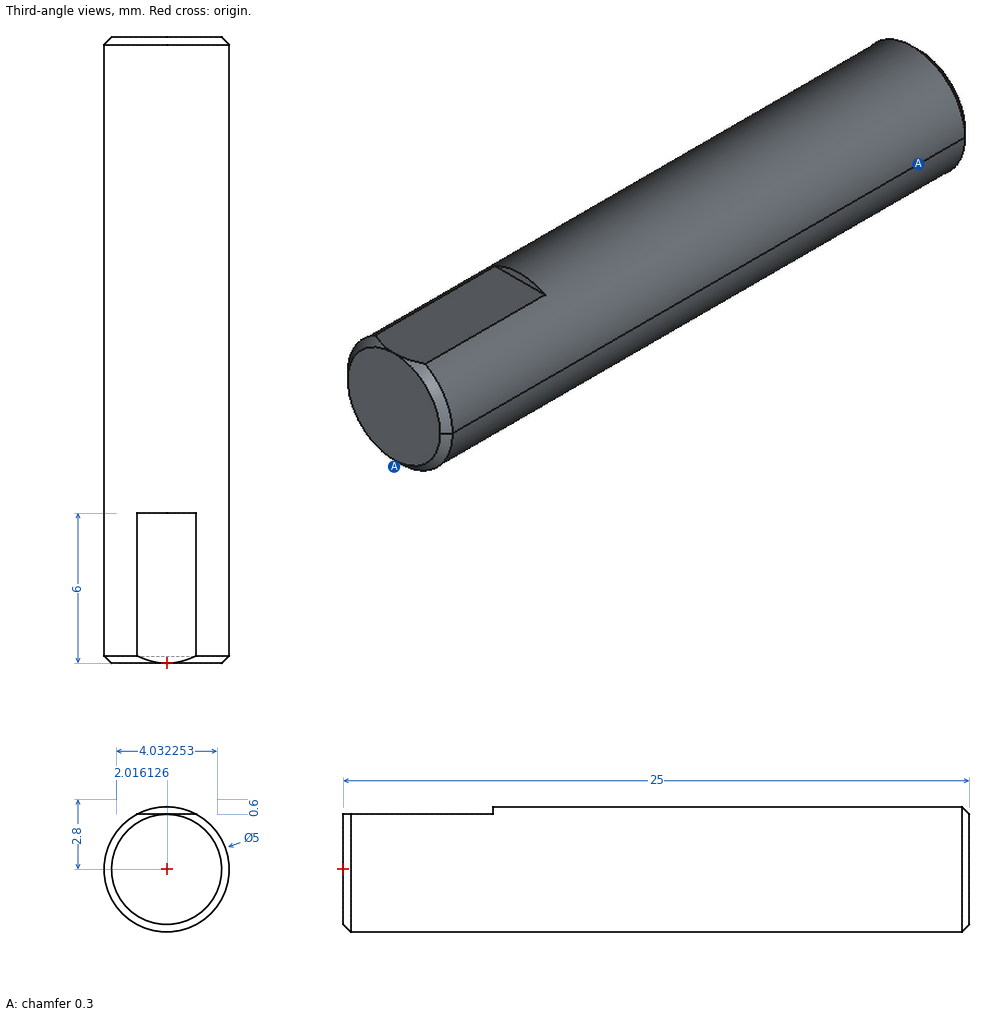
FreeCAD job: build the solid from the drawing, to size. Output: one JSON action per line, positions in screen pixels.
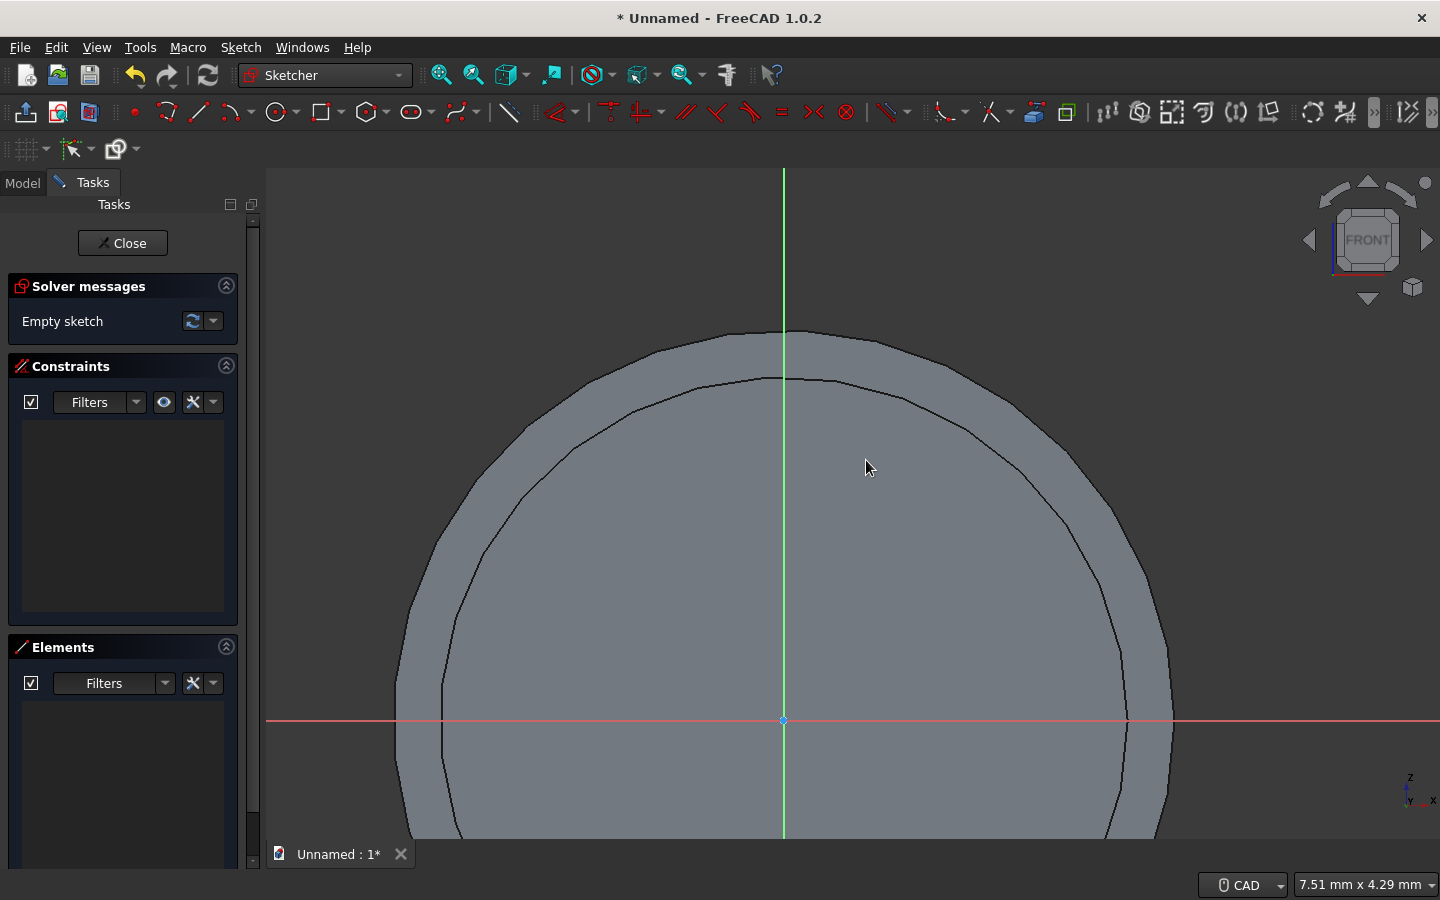
{"action": "left_click", "coordinate": [322, 112]}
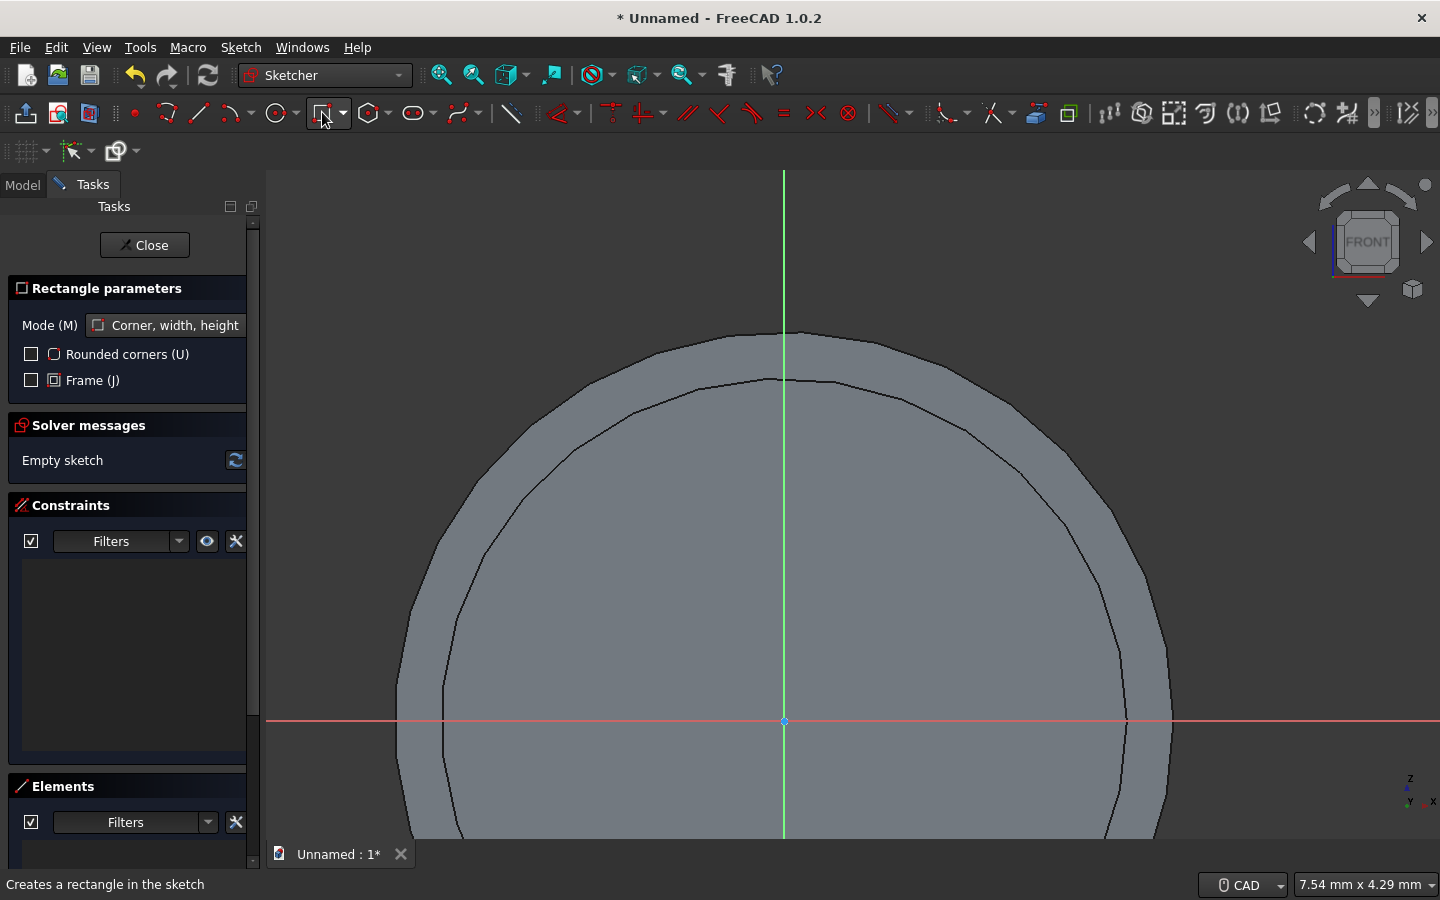
{"action": "left_click", "coordinate": [470, 285]}
{"action": "mouse_move", "coordinate": [1098, 379]}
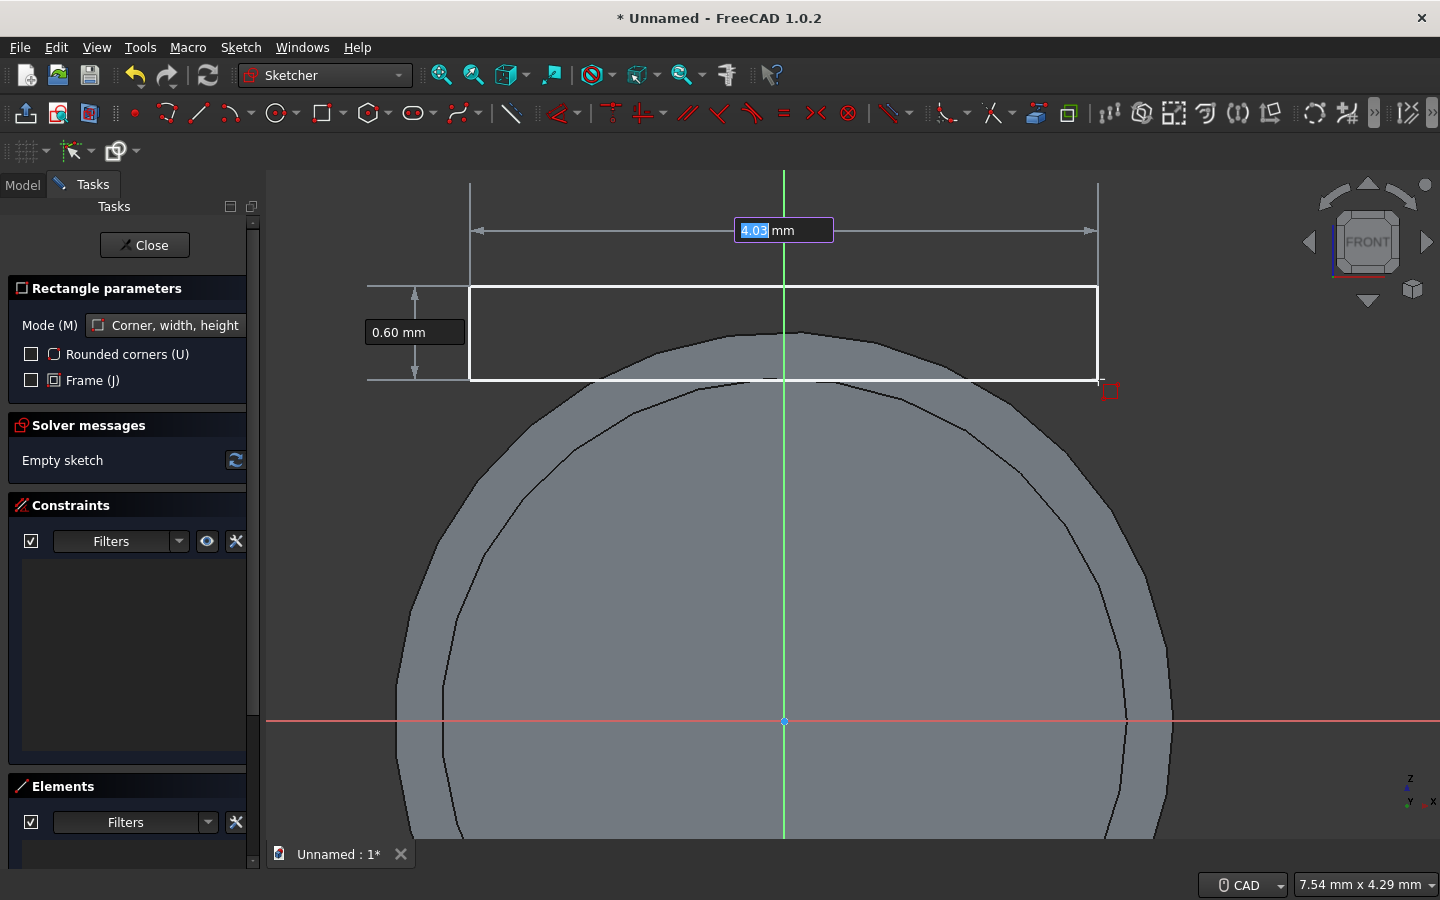
{"action": "type", "text": "4.032253"}
{"action": "key", "text": "Tab"}
{"action": "type", "text": "0.6"}
{"action": "key", "text": "Return"}
{"action": "key", "text": "Escape"}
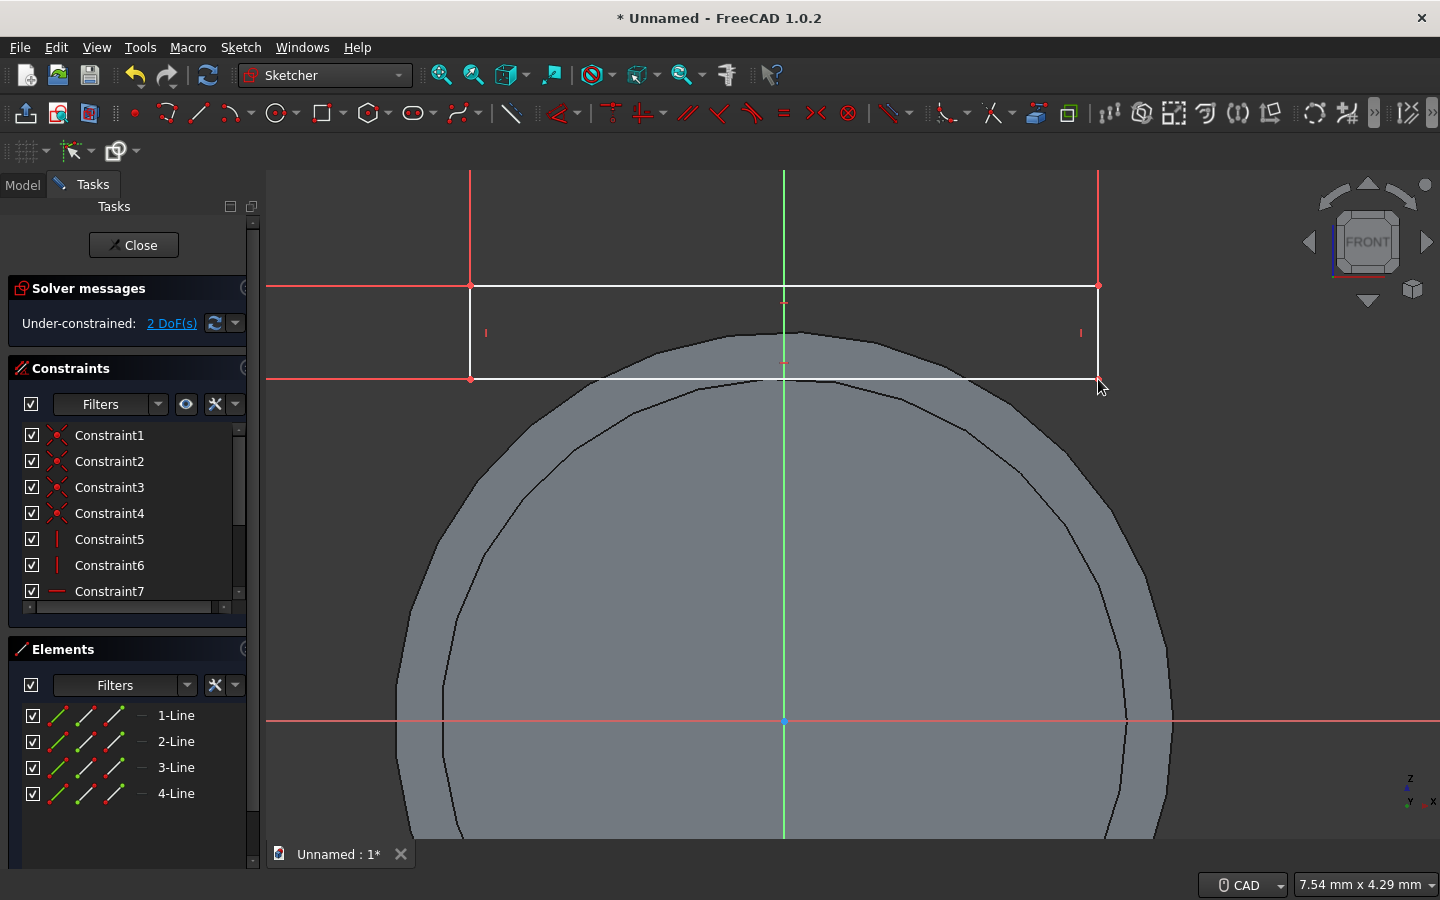
{"action": "left_click", "coordinate": [470, 286]}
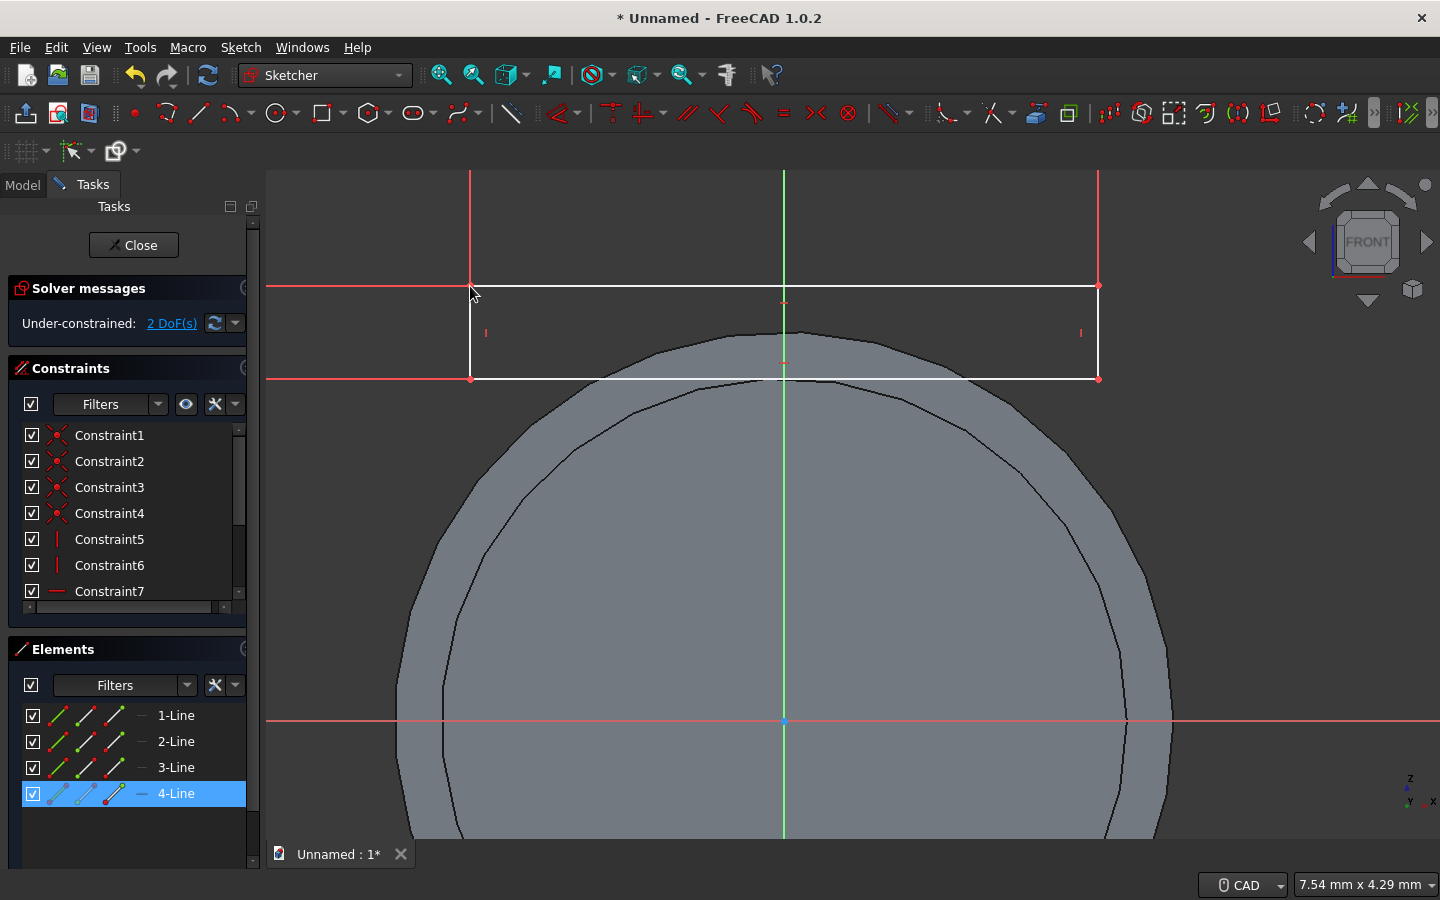
{"action": "key", "text": "i"}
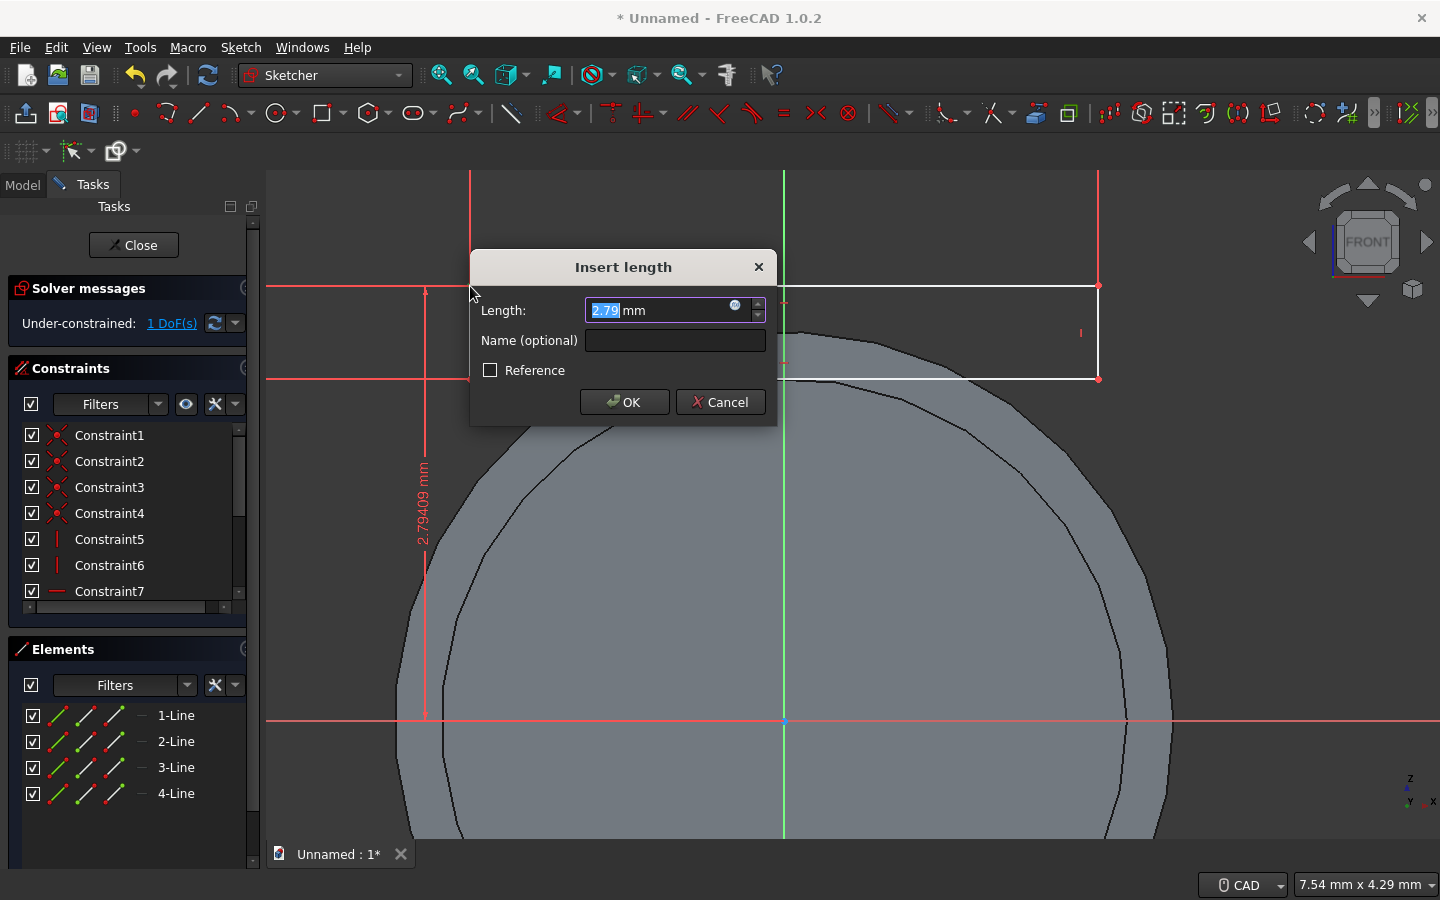
{"action": "type", "text": "2.8"}
{"action": "key", "text": "Return"}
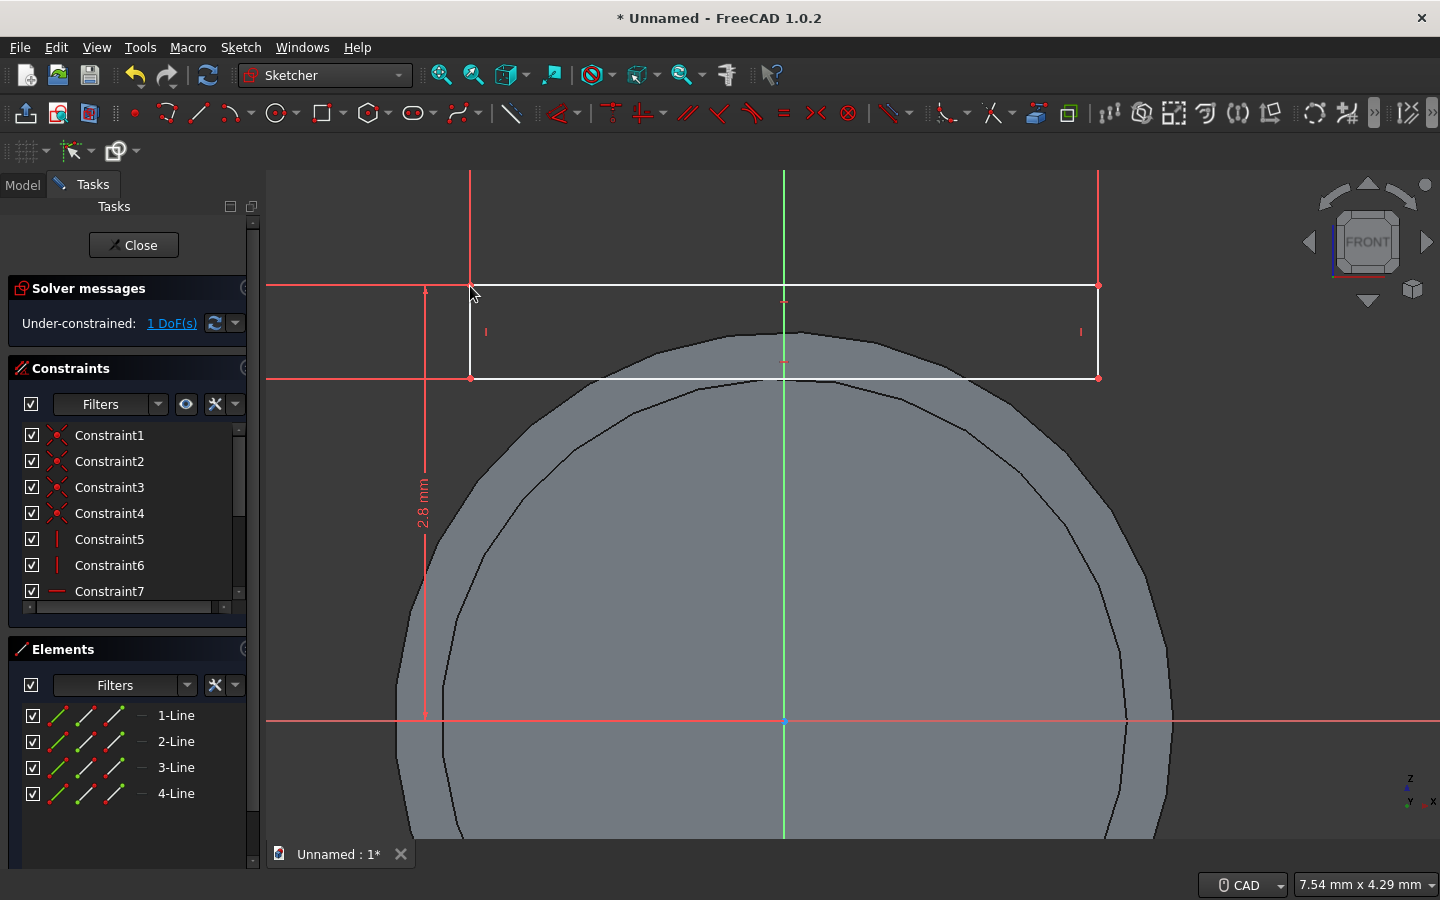
{"action": "left_click", "coordinate": [470, 285]}